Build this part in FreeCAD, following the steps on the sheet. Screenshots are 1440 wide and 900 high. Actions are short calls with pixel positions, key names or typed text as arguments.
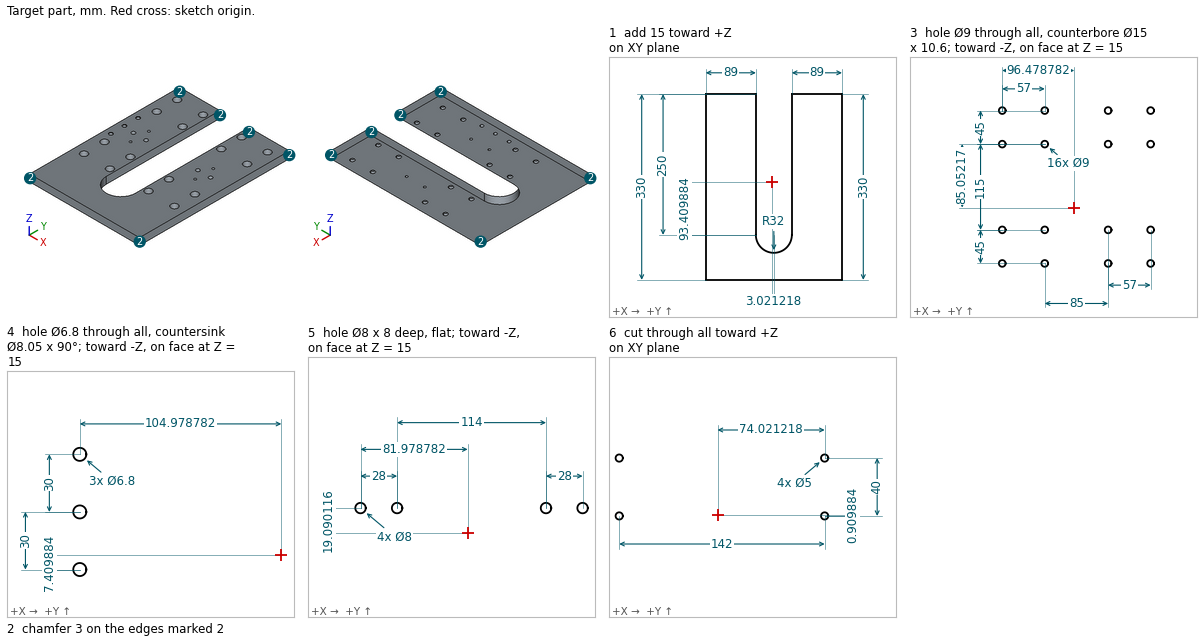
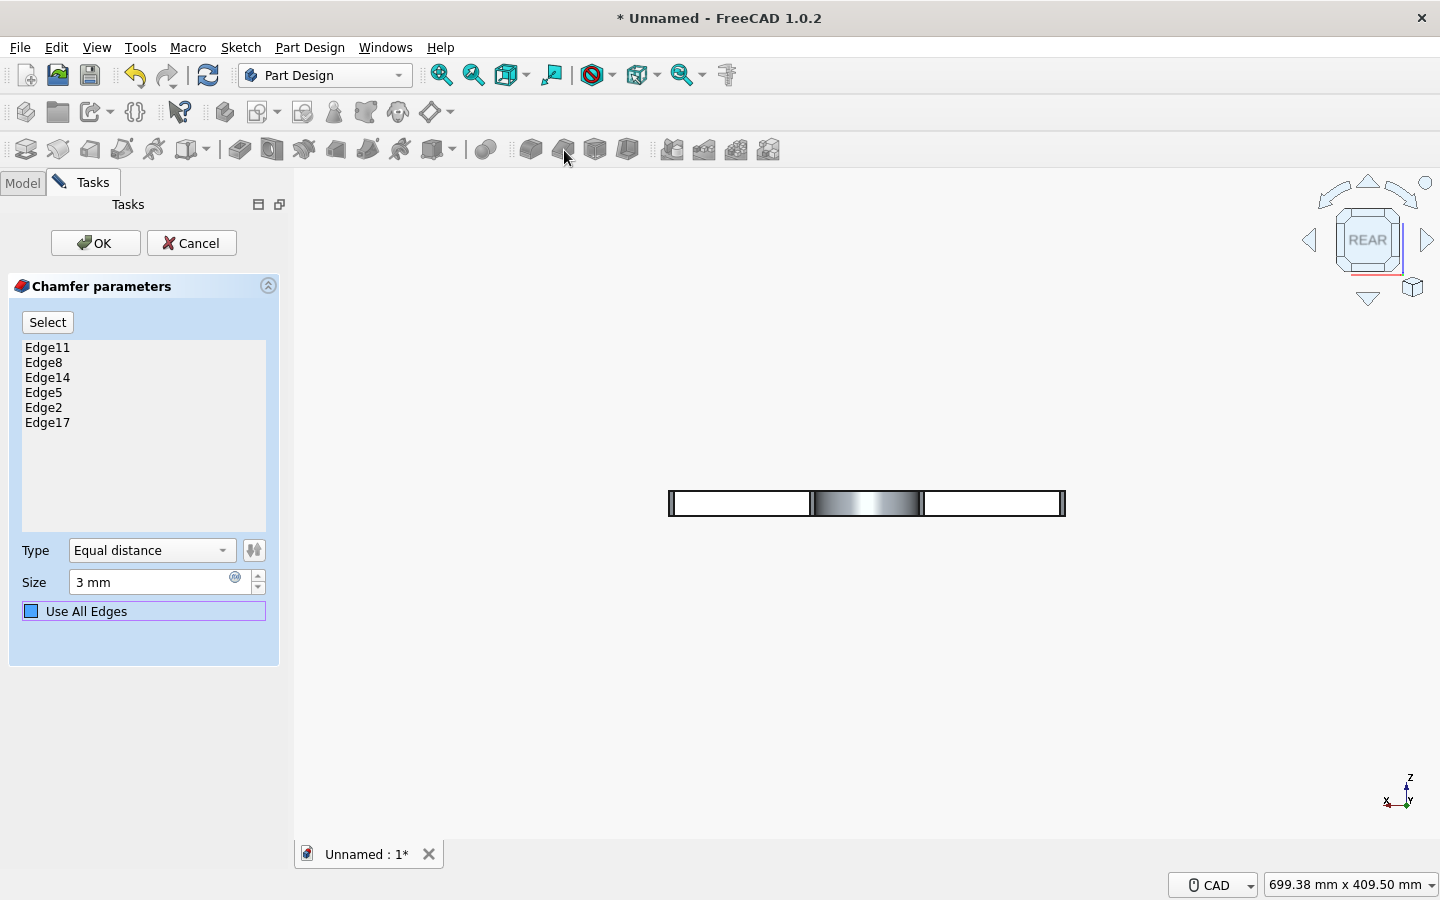
click(96, 243)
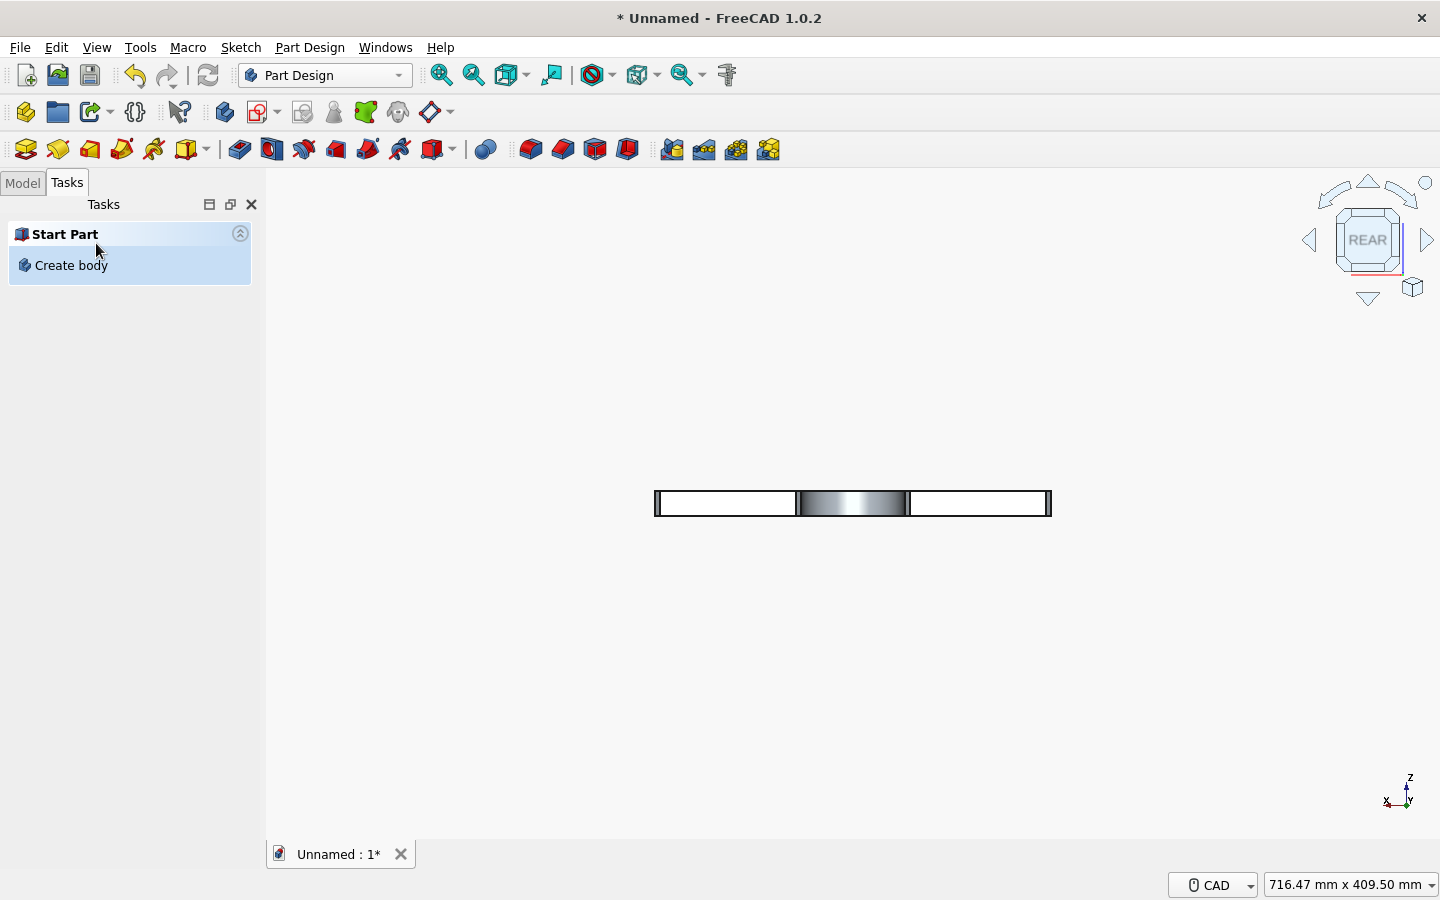
click(442, 76)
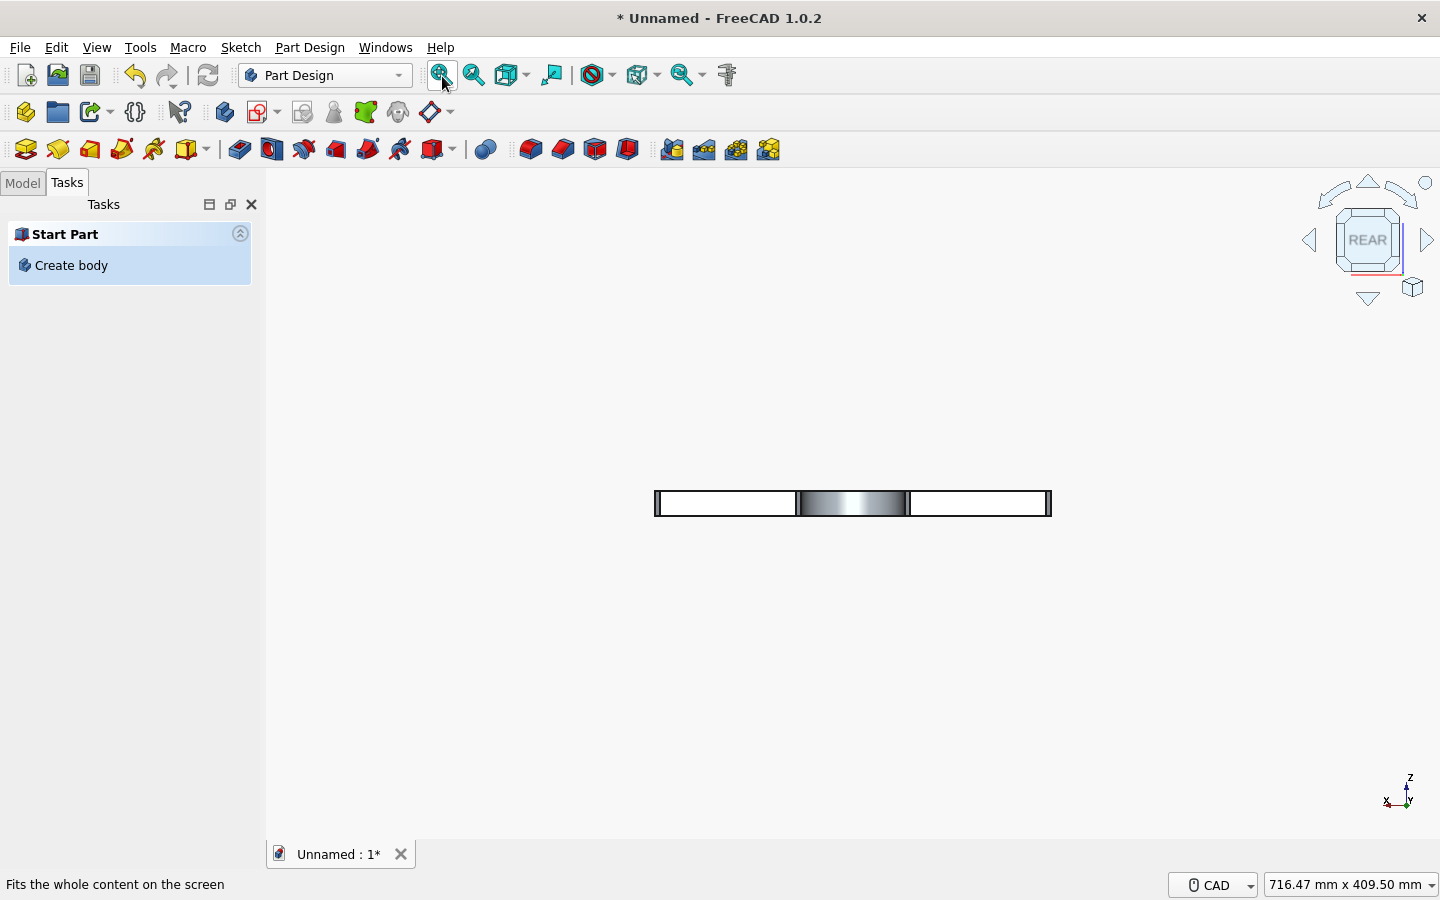
key(0)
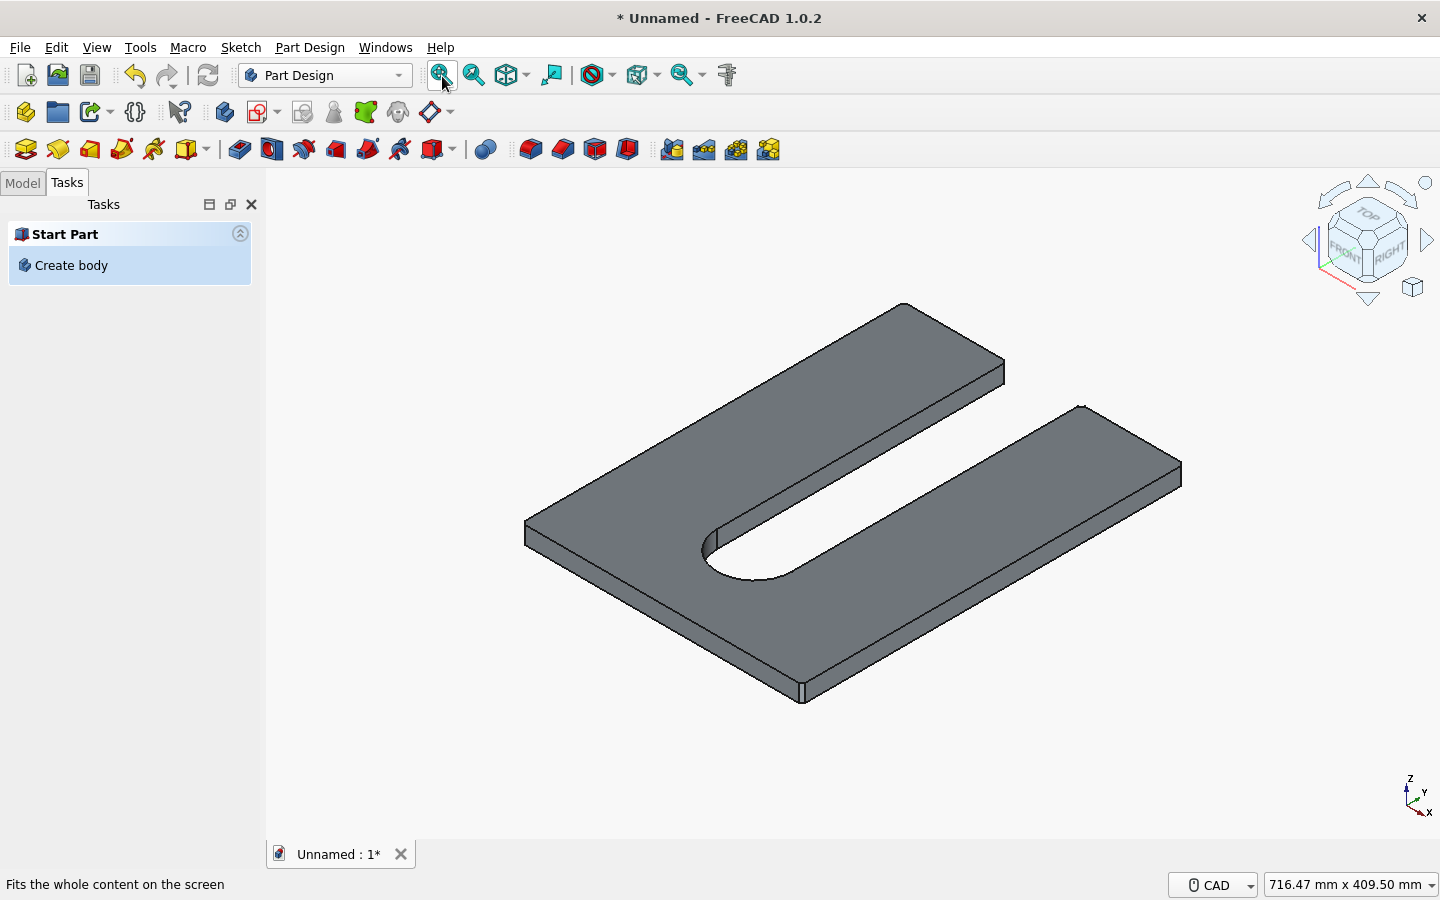
click(824, 602)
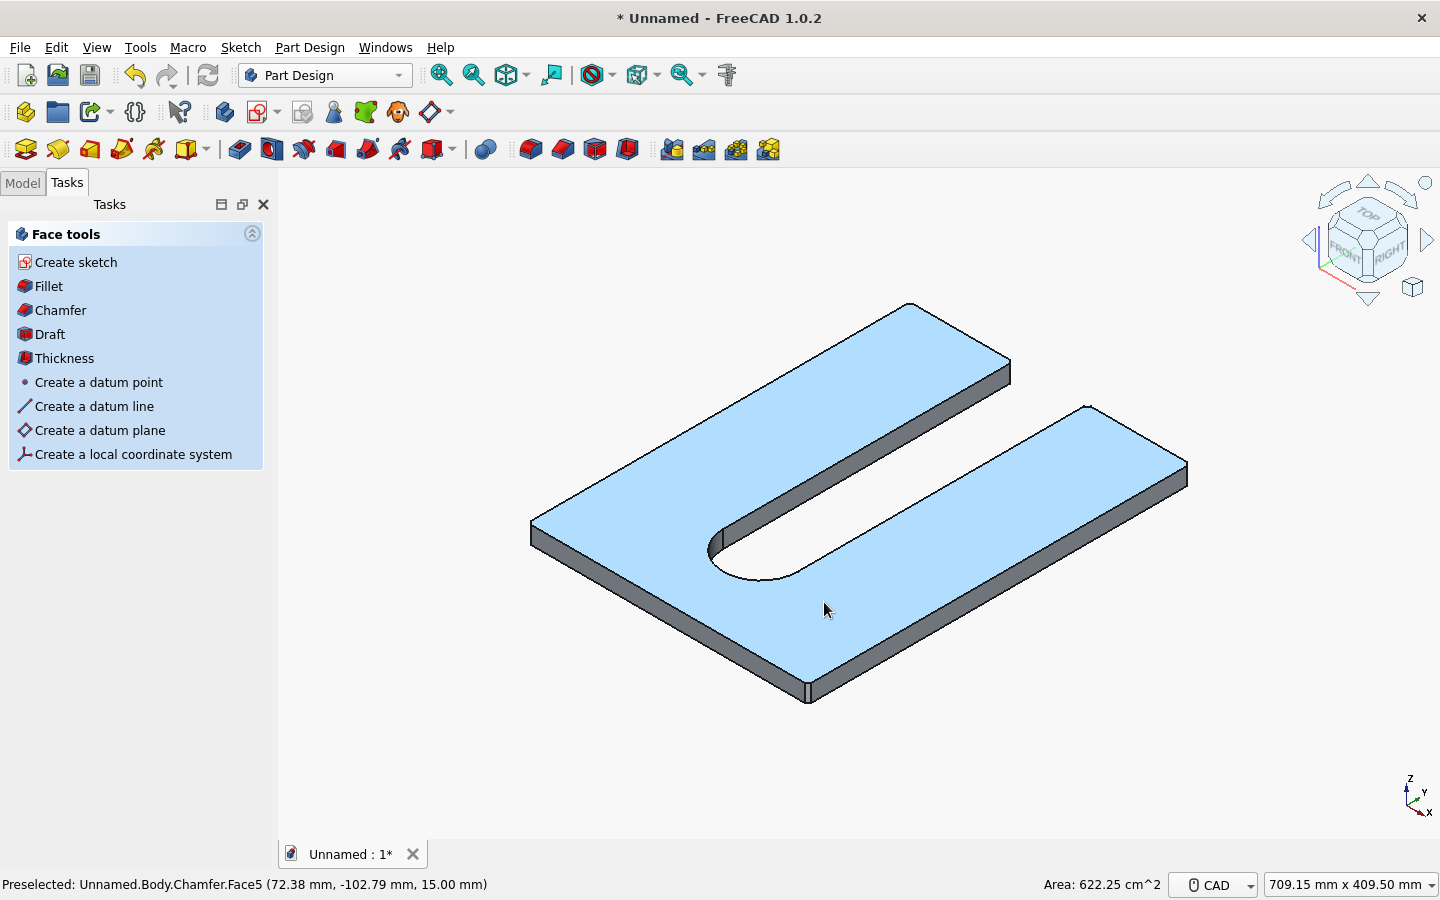
click(258, 112)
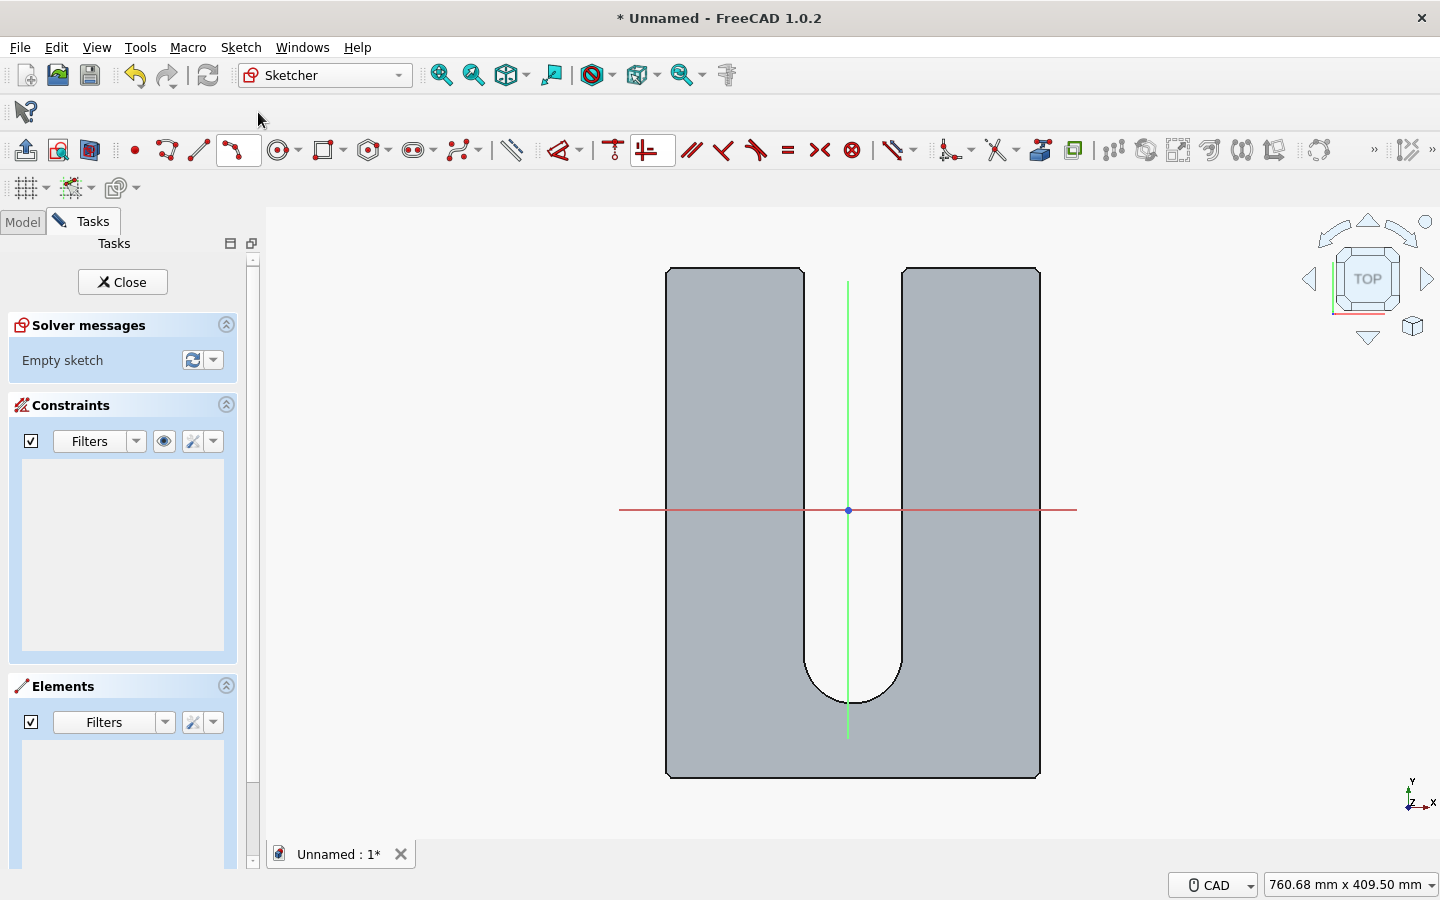
click(278, 150)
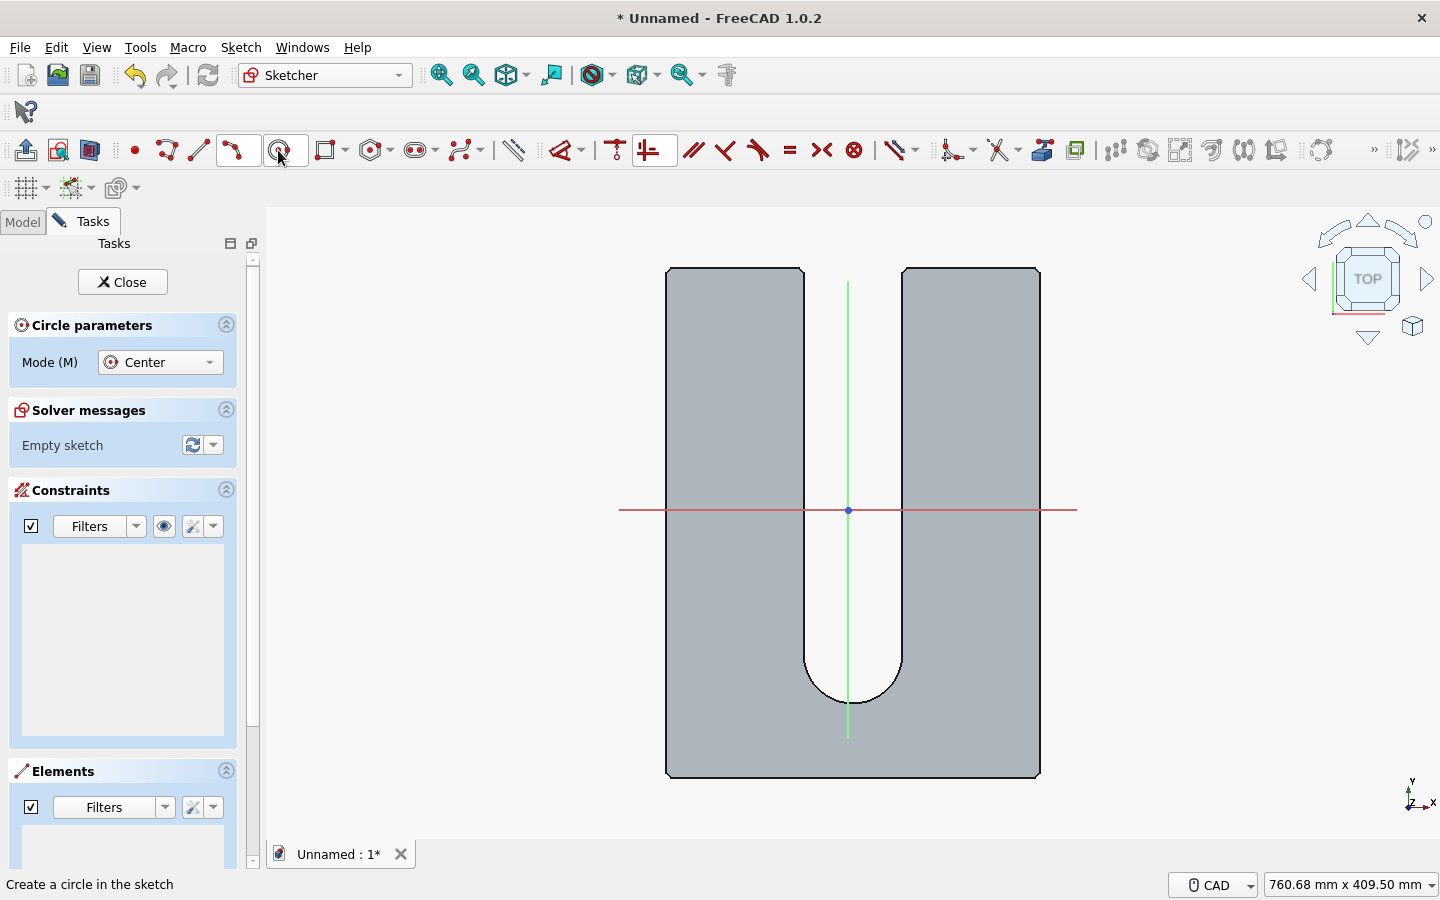
scroll(699, 309, up, 6)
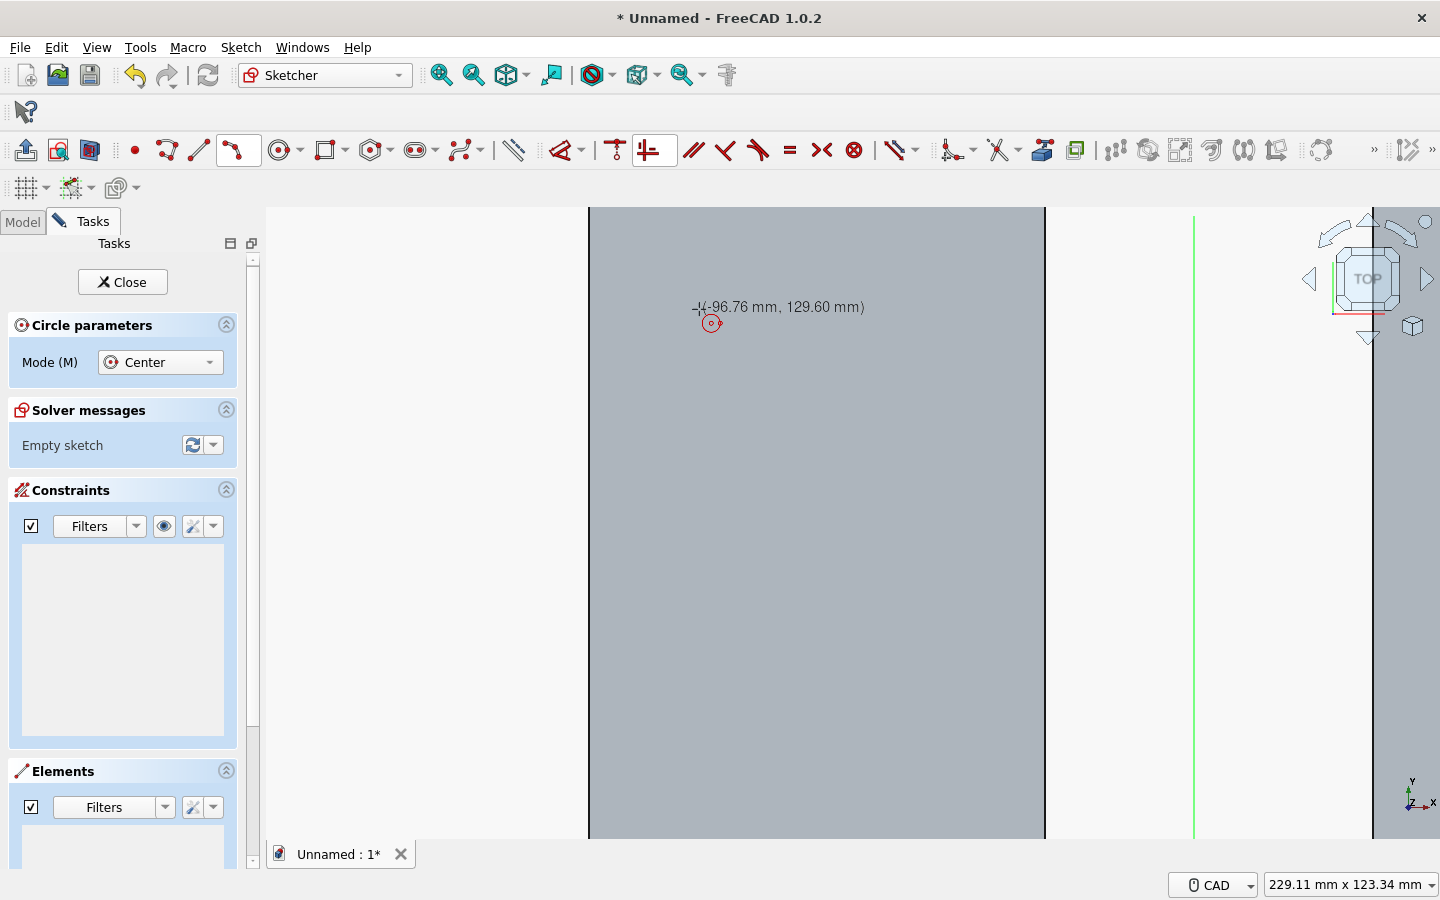
click(700, 310)
move(716, 293)